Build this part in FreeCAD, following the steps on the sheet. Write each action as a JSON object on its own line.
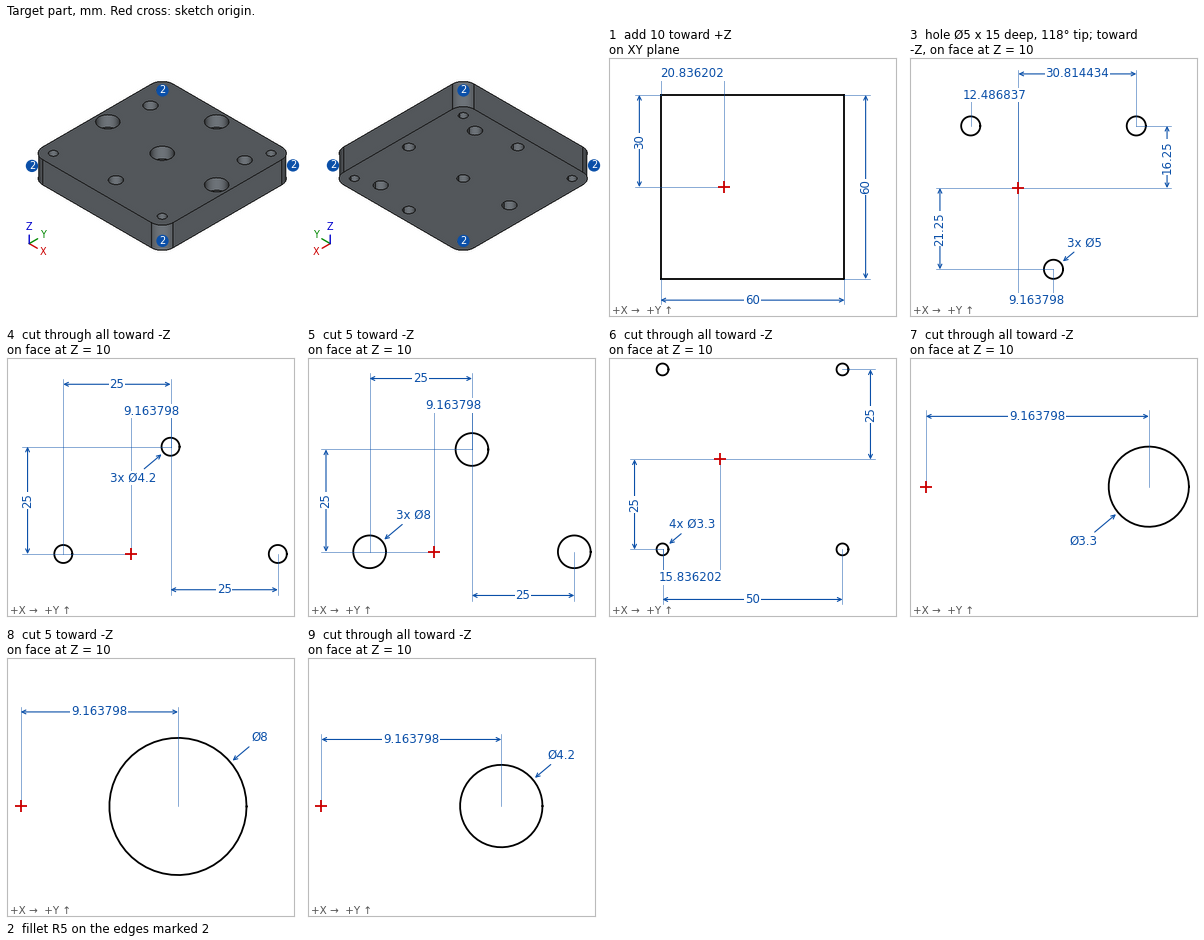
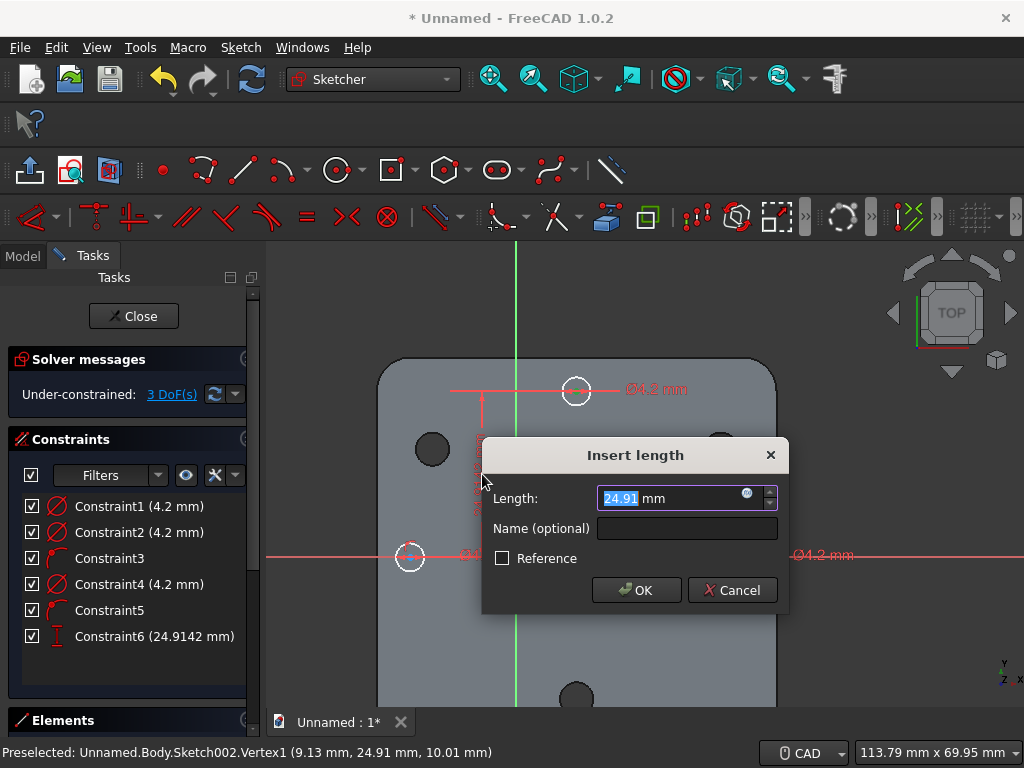
{"action": "type", "text": "25"}
{"action": "key", "text": "Return"}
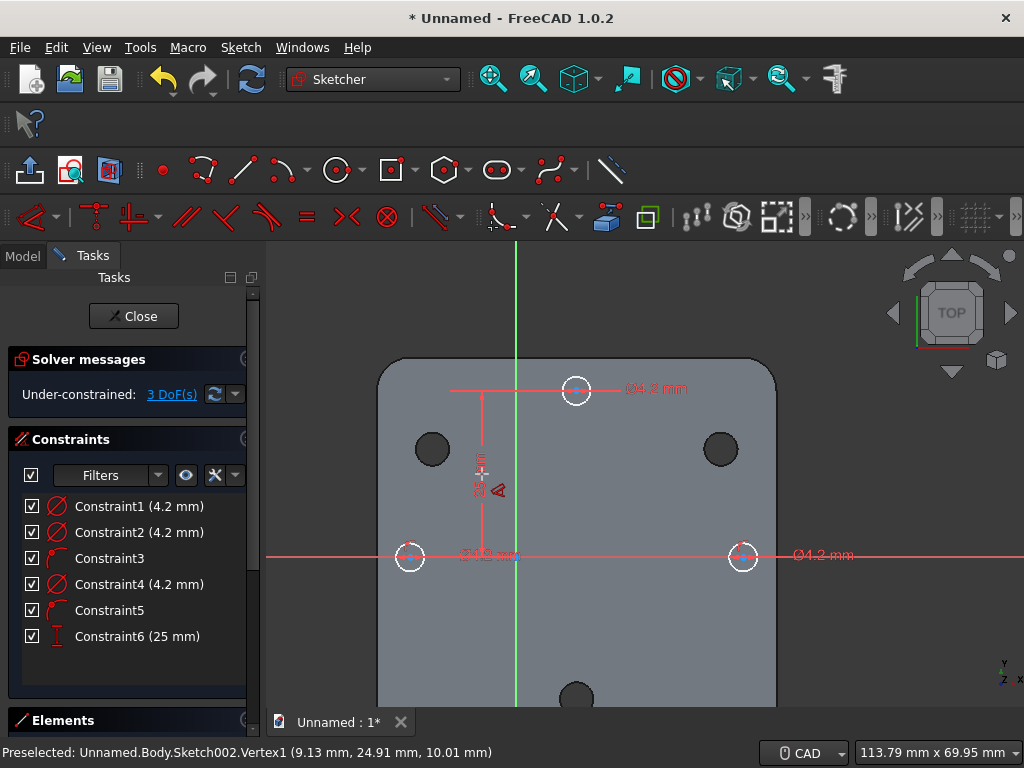
{"action": "left_click", "coordinate": [576, 391]}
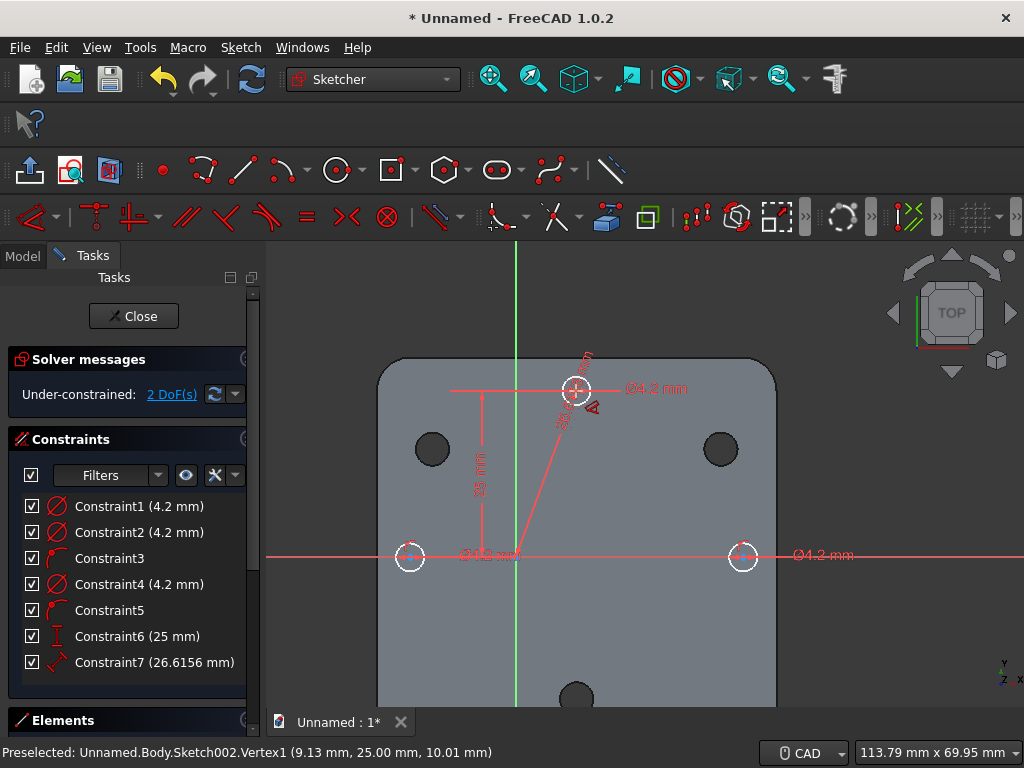
{"action": "left_click", "coordinate": [743, 557]}
{"action": "left_click", "coordinate": [660, 591]}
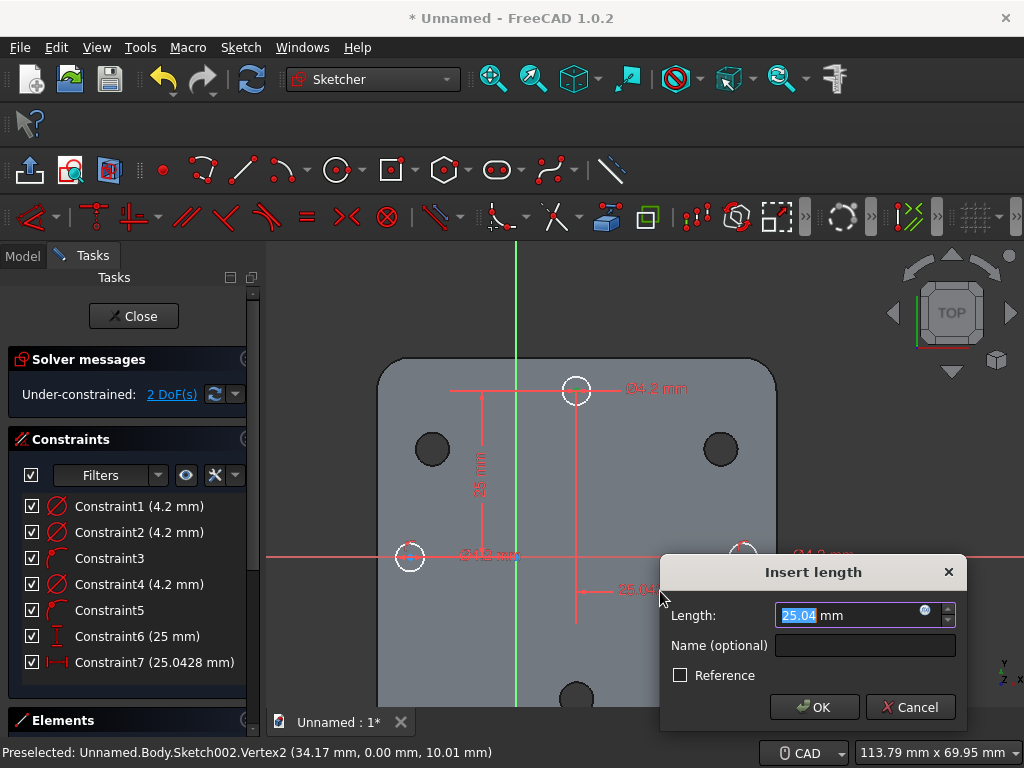
{"action": "type", "text": "25"}
{"action": "key", "text": "Return"}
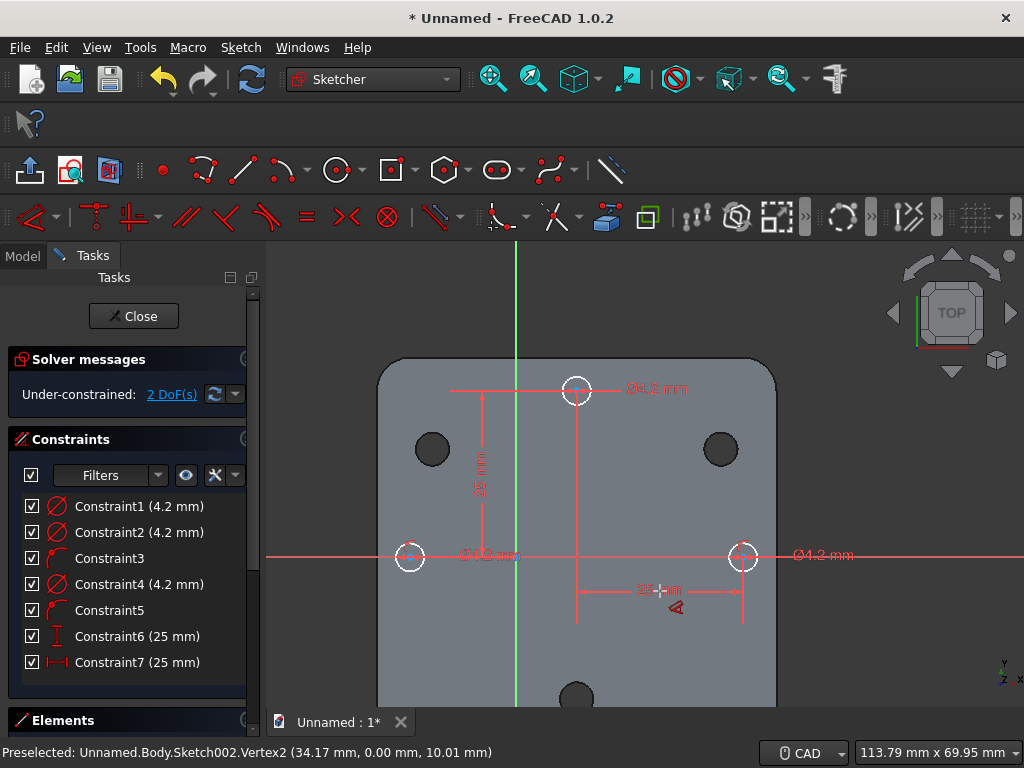
{"action": "left_click", "coordinate": [577, 391]}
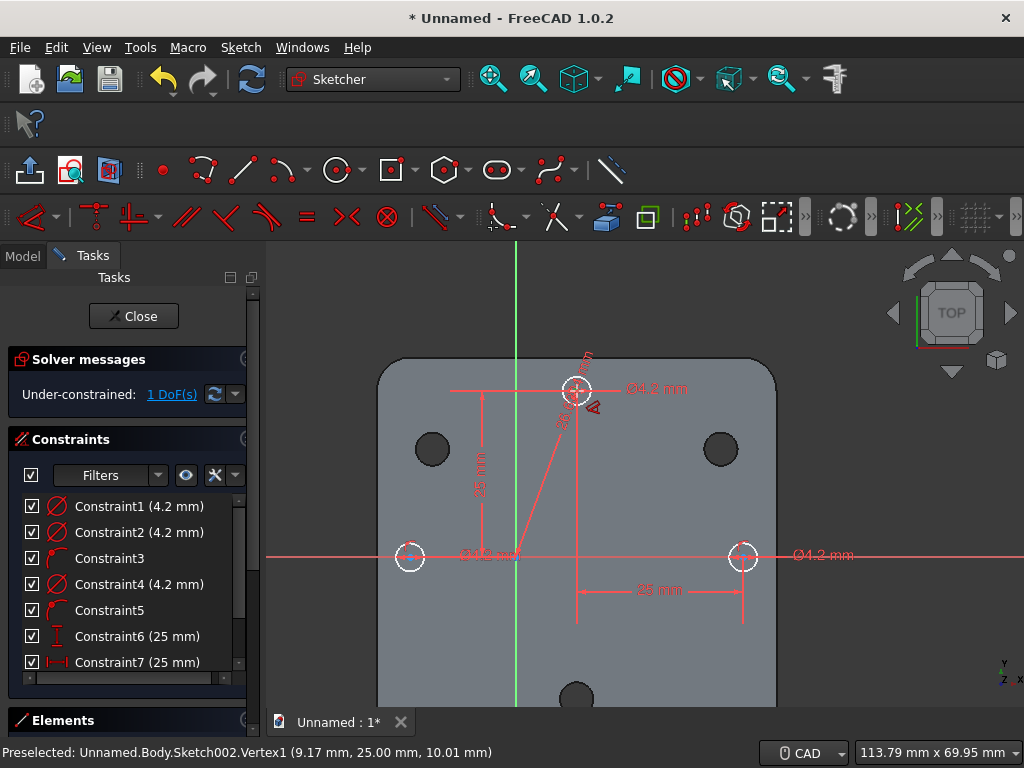
{"action": "left_click", "coordinate": [410, 557]}
{"action": "left_click", "coordinate": [493, 591]}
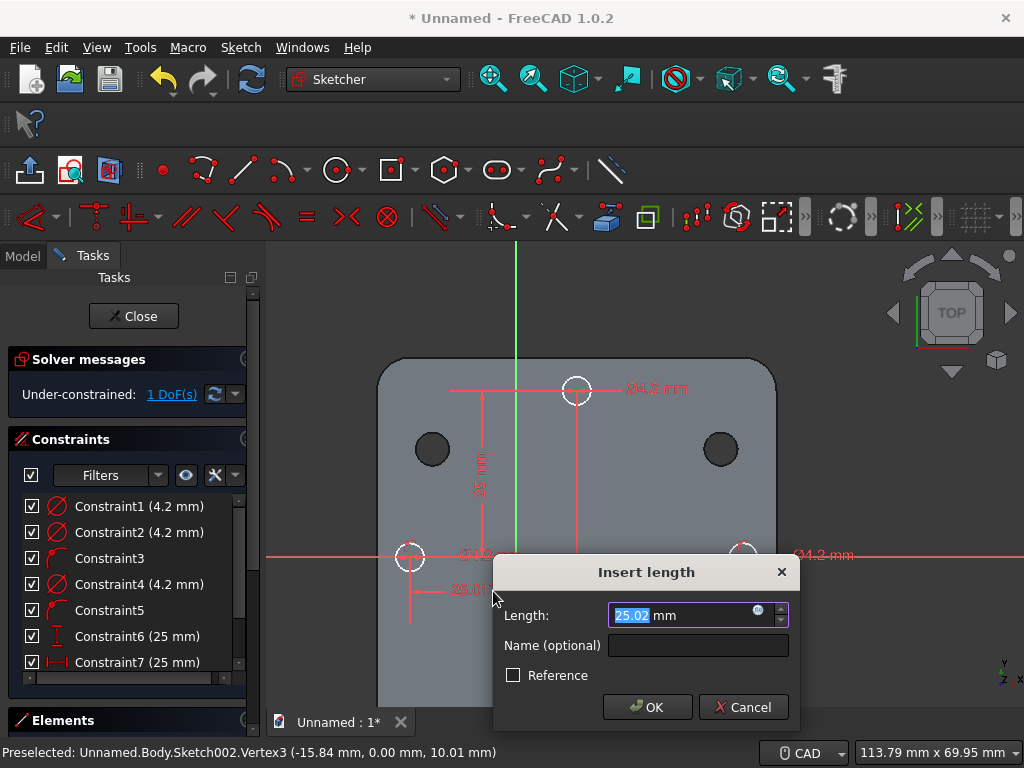
{"action": "type", "text": "25"}
{"action": "key", "text": "Return"}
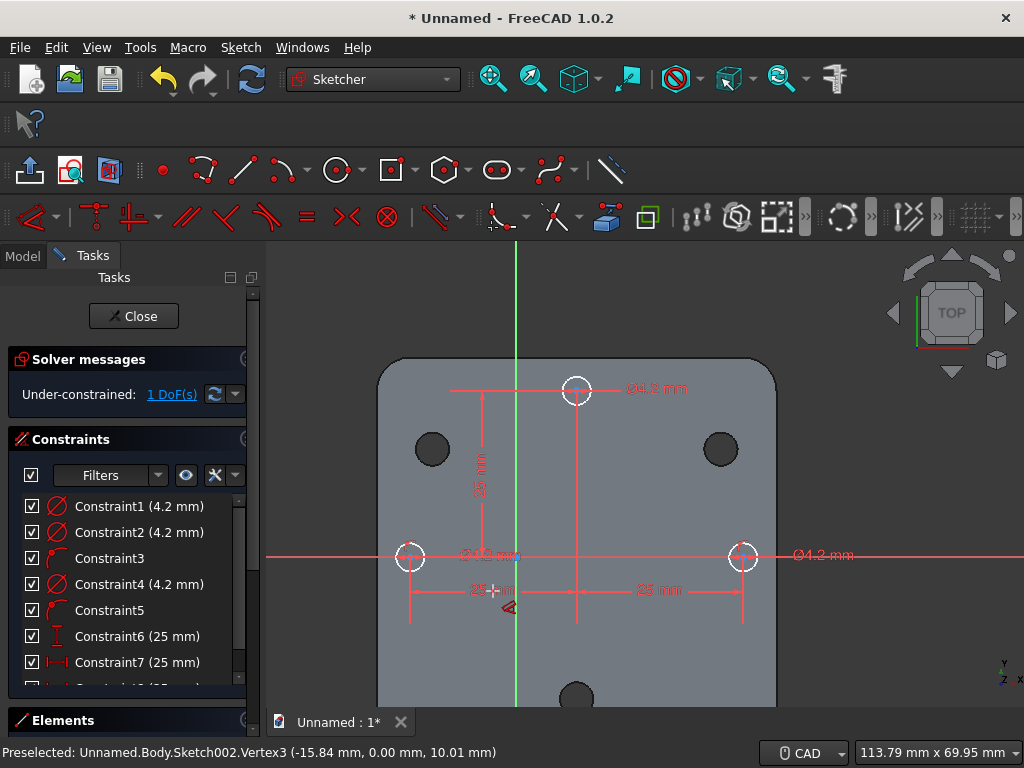
{"action": "left_click", "coordinate": [577, 391]}
{"action": "left_click", "coordinate": [568, 591]}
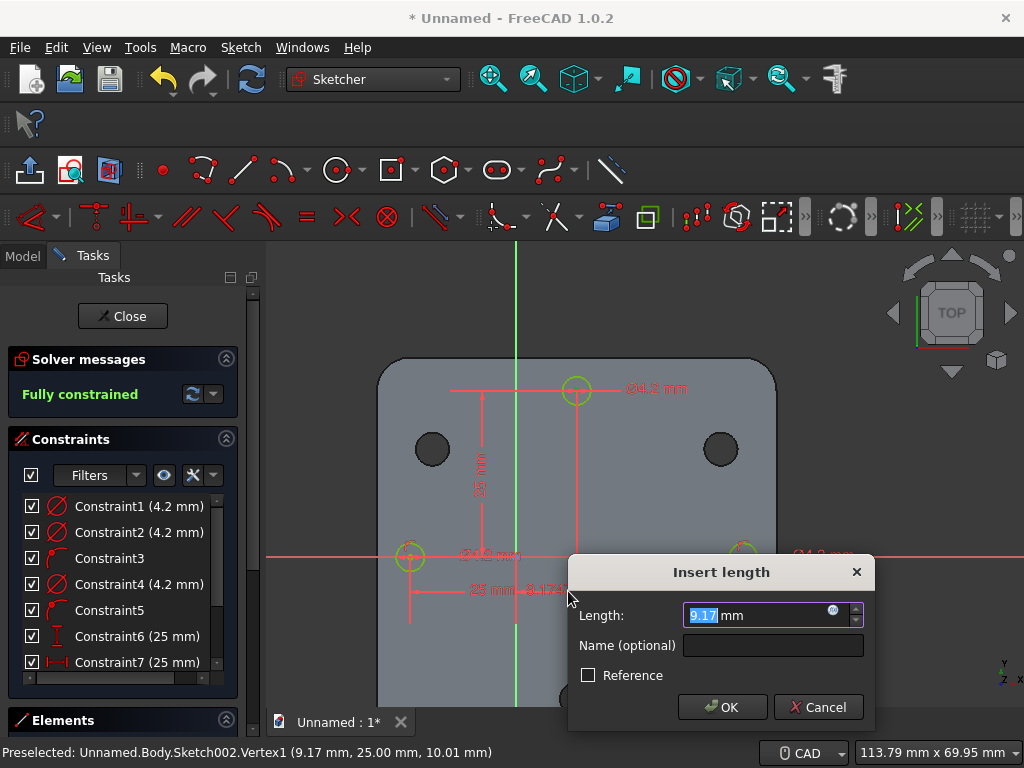
{"action": "type", "text": "9.163798"}
{"action": "key", "text": "Return"}
{"action": "key", "text": "Escape"}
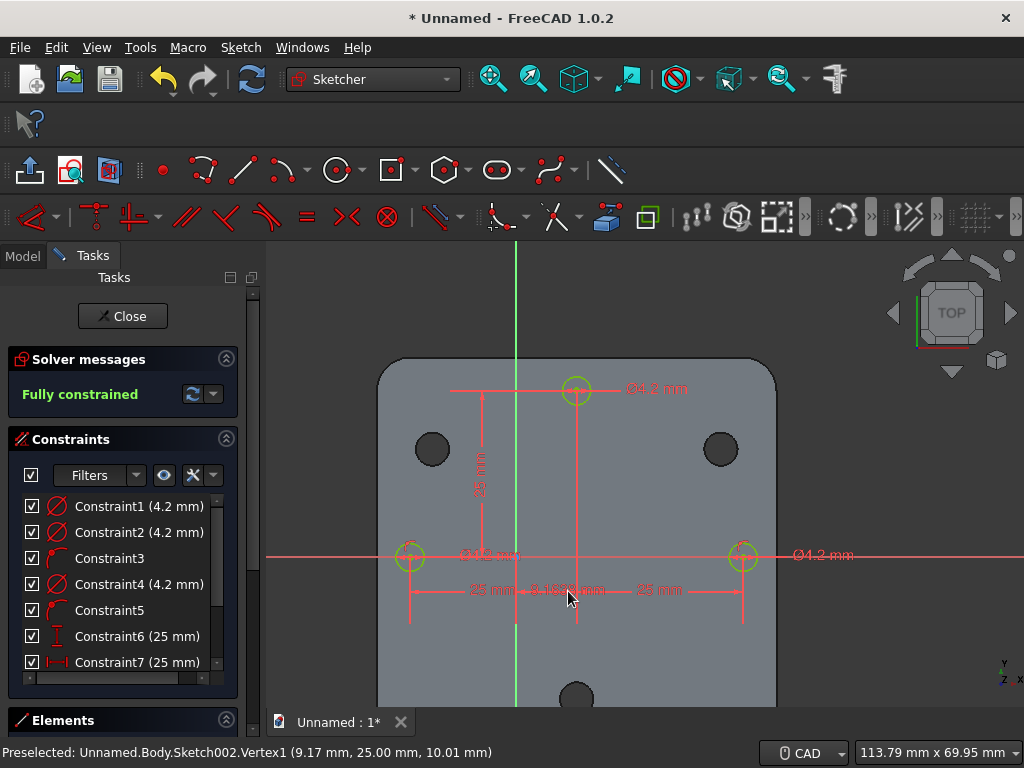
{"action": "left_click", "coordinate": [123, 316]}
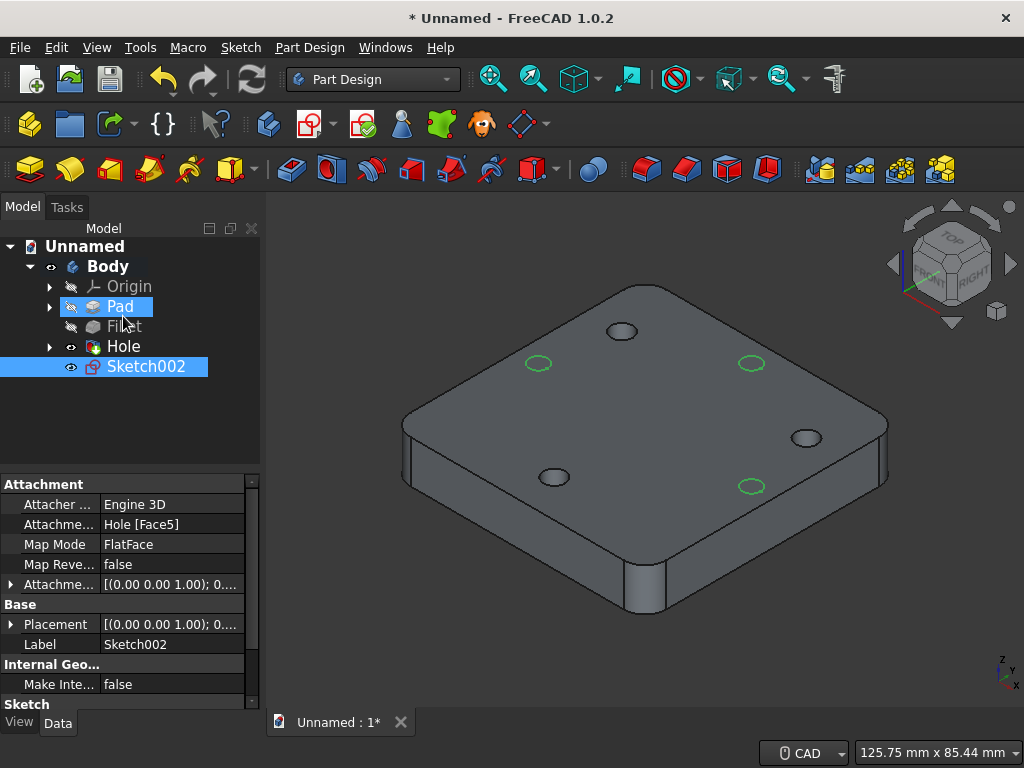
{"action": "left_click", "coordinate": [292, 170]}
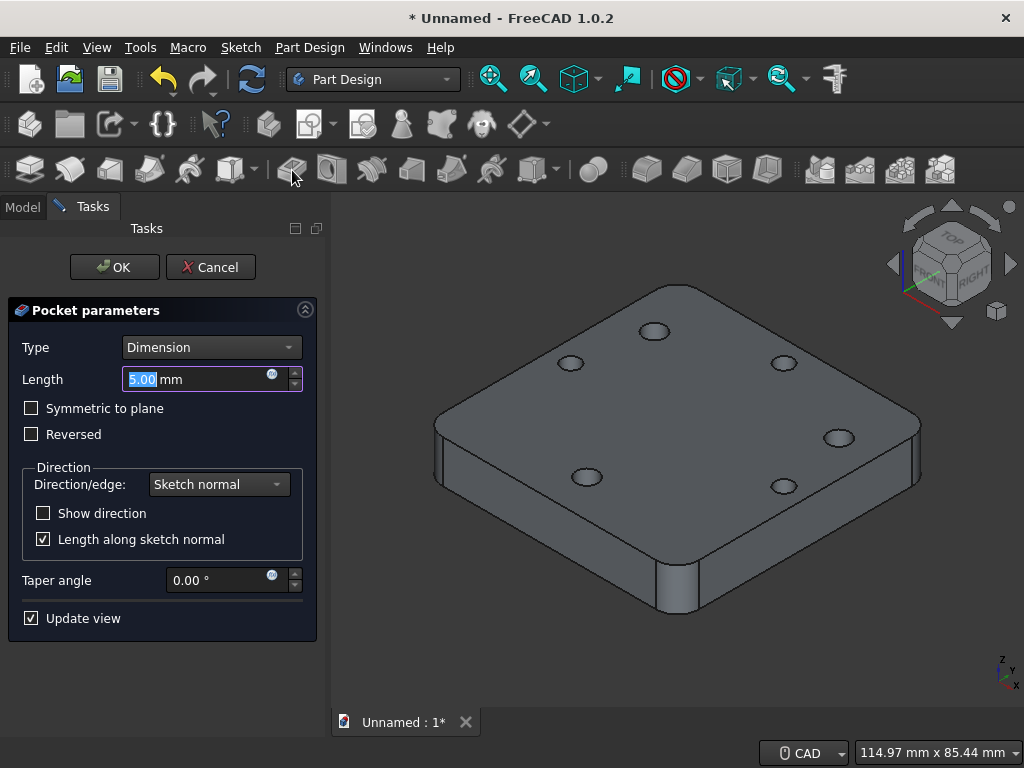
{"action": "left_click", "coordinate": [212, 348]}